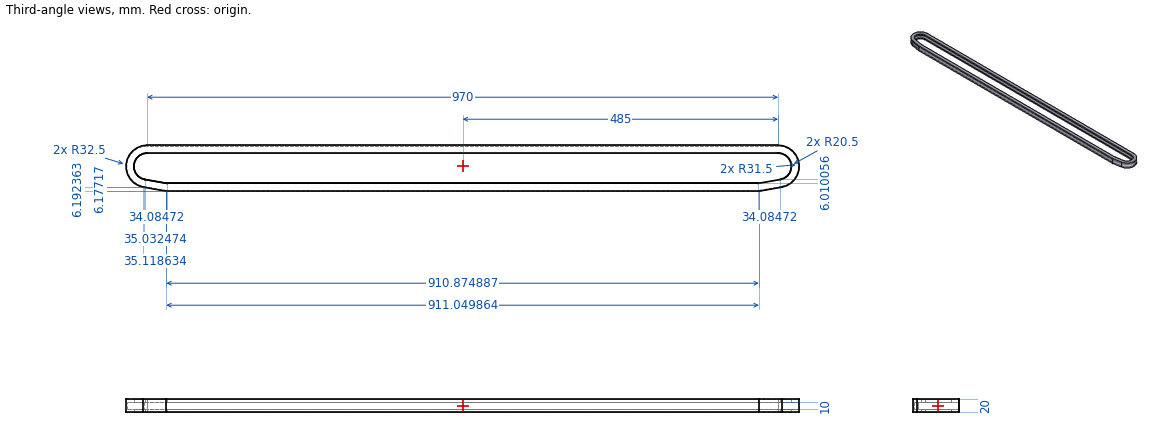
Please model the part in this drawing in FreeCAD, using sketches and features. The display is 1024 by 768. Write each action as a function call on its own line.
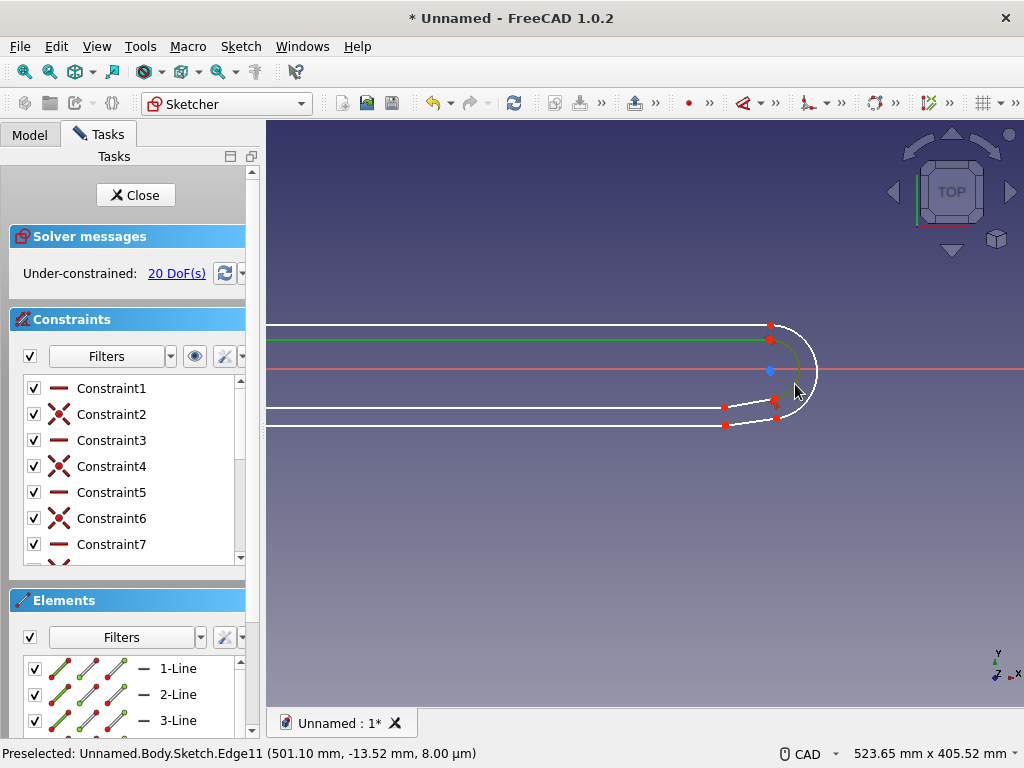
key(t)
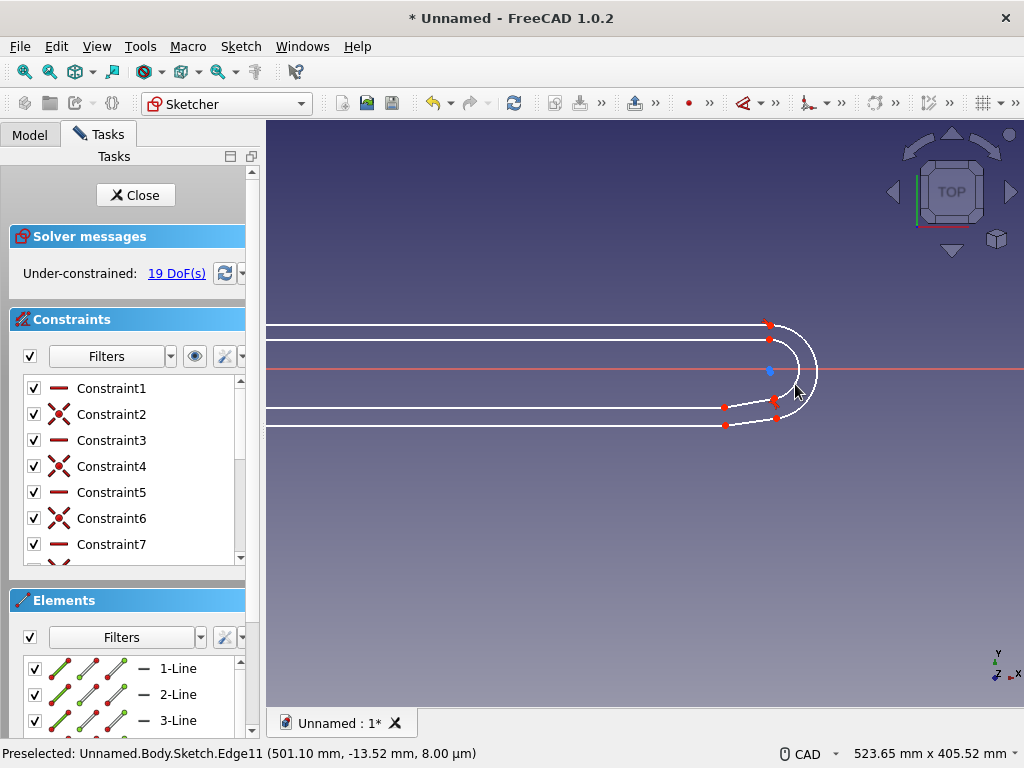
click(348, 340)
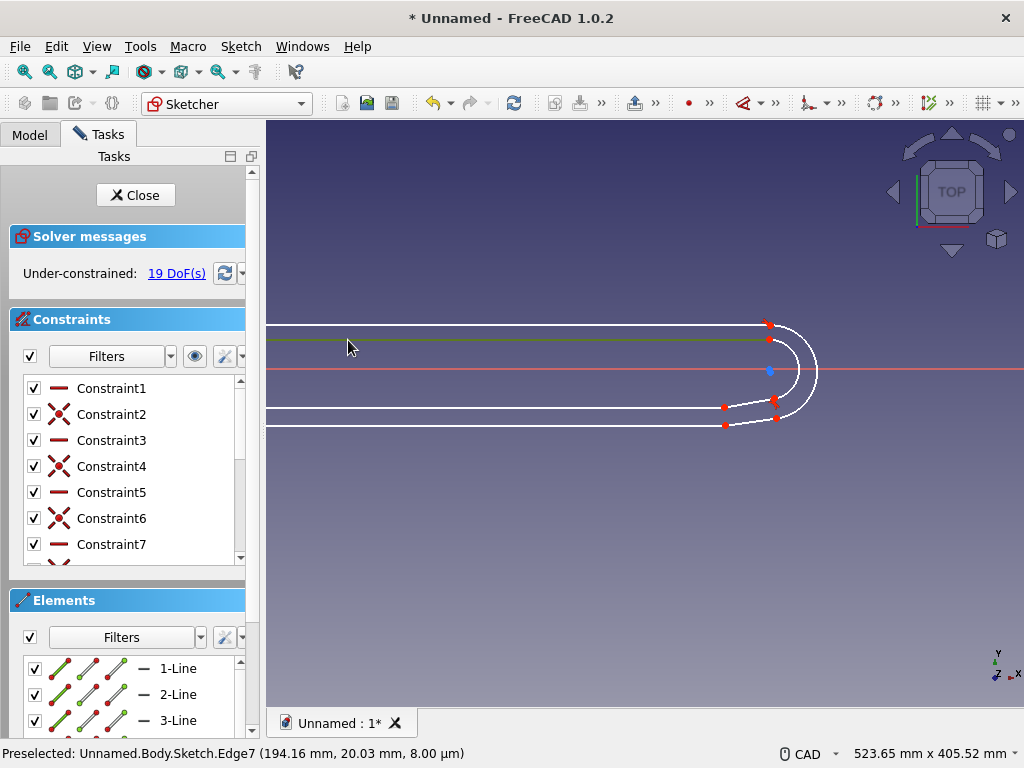
scroll(743, 427, down, 7)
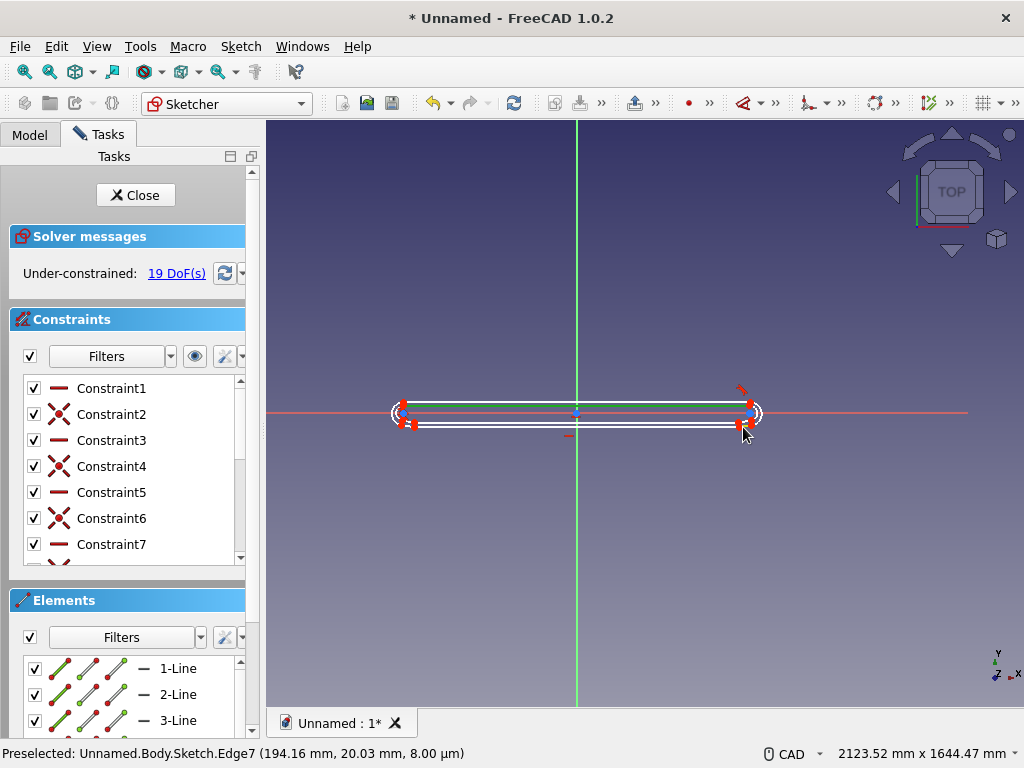
scroll(398, 409, up, 7)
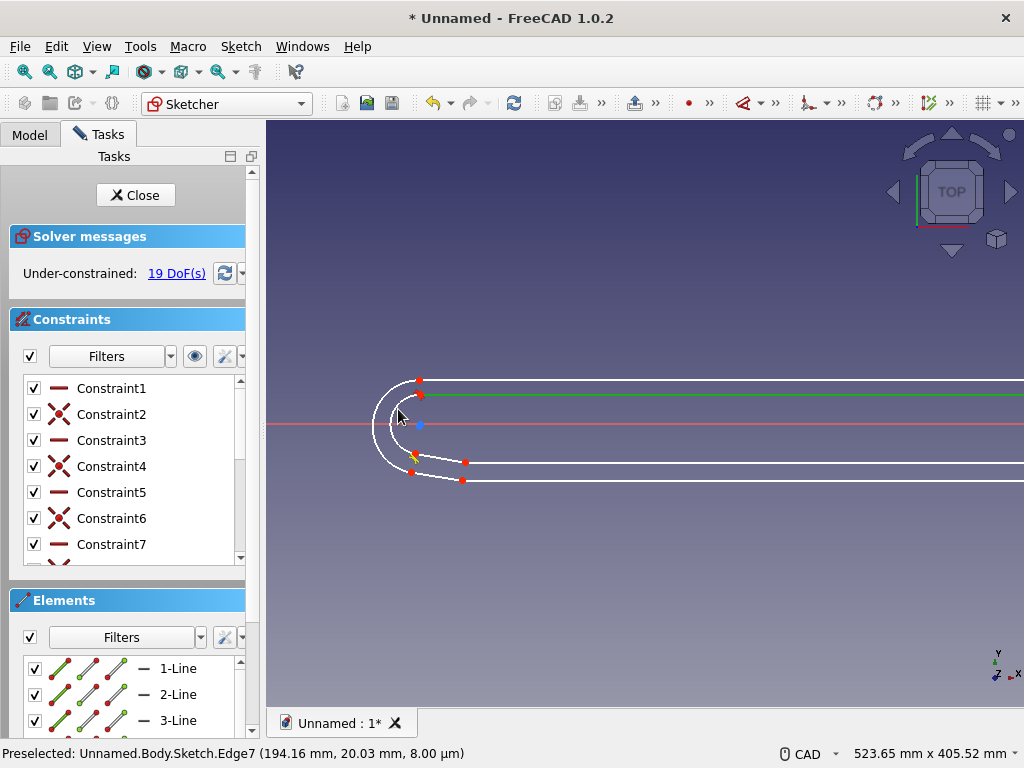
click(397, 406)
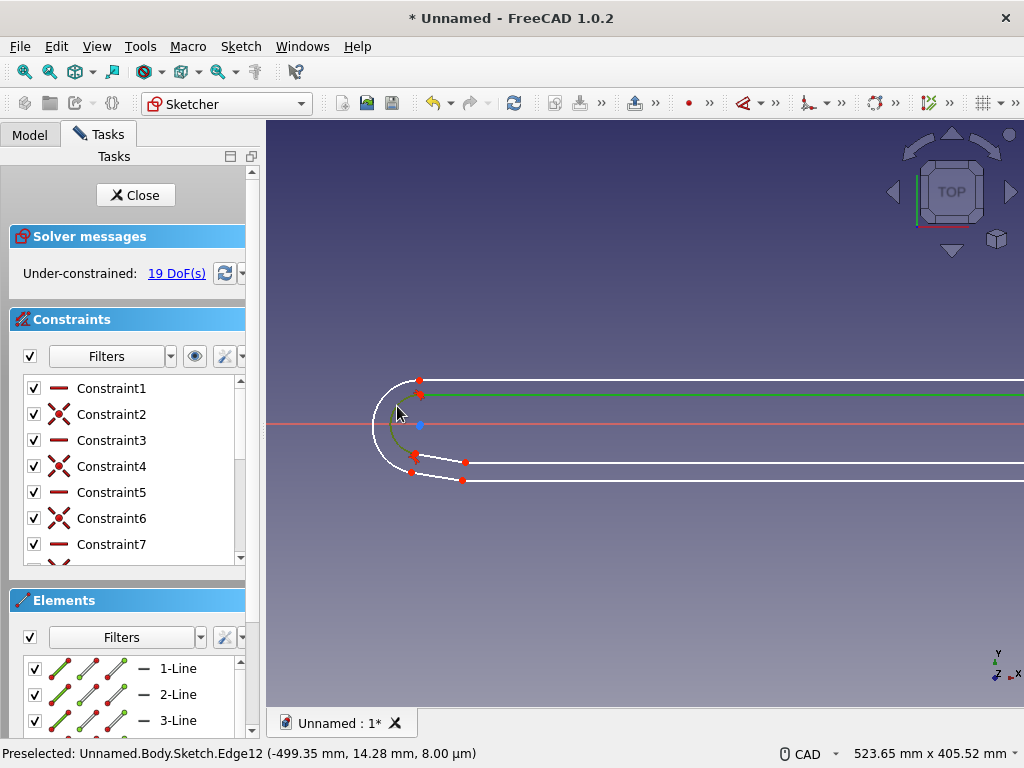
key(t)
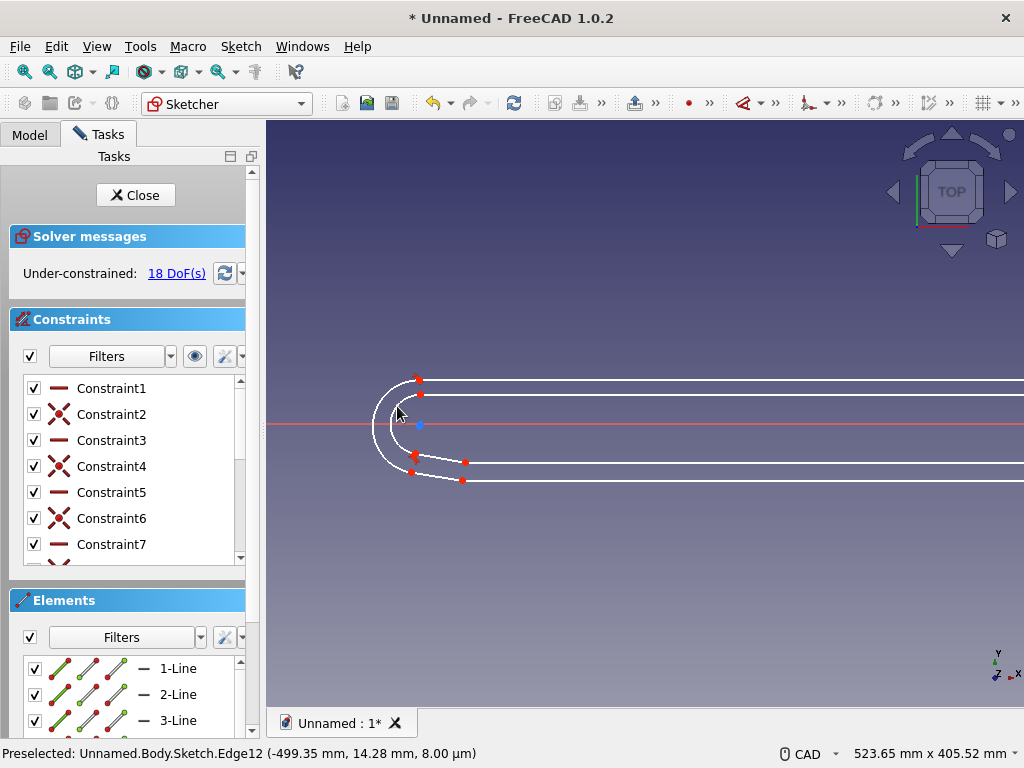
scroll(398, 409, down, 7)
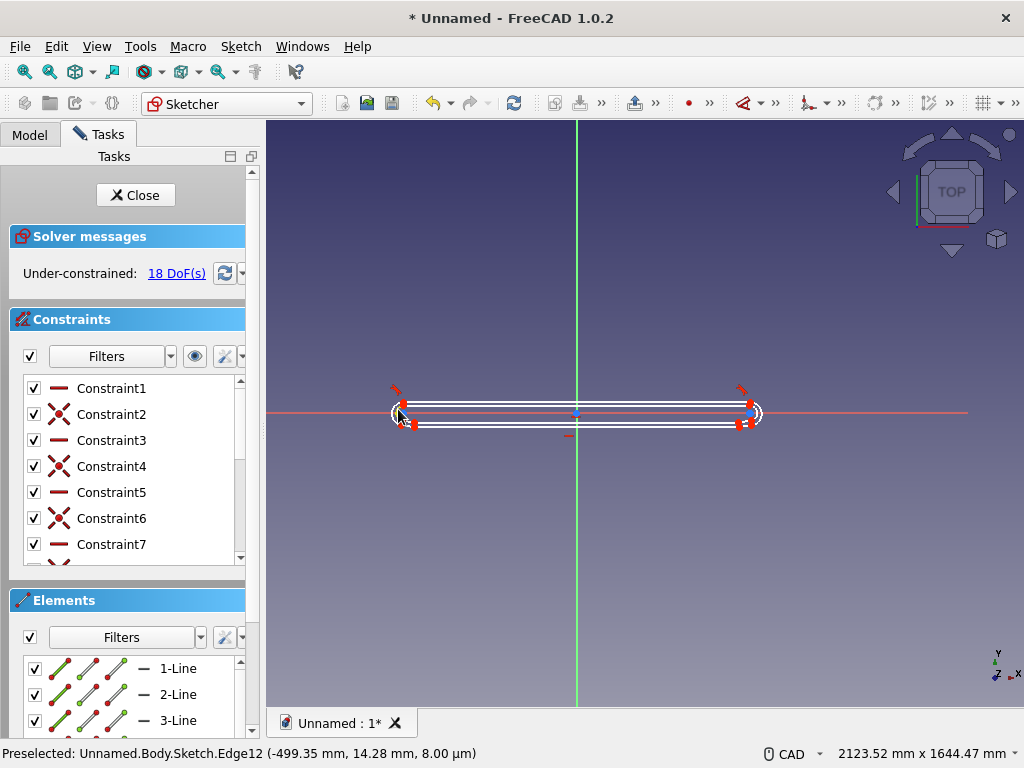
scroll(748, 421, up, 7)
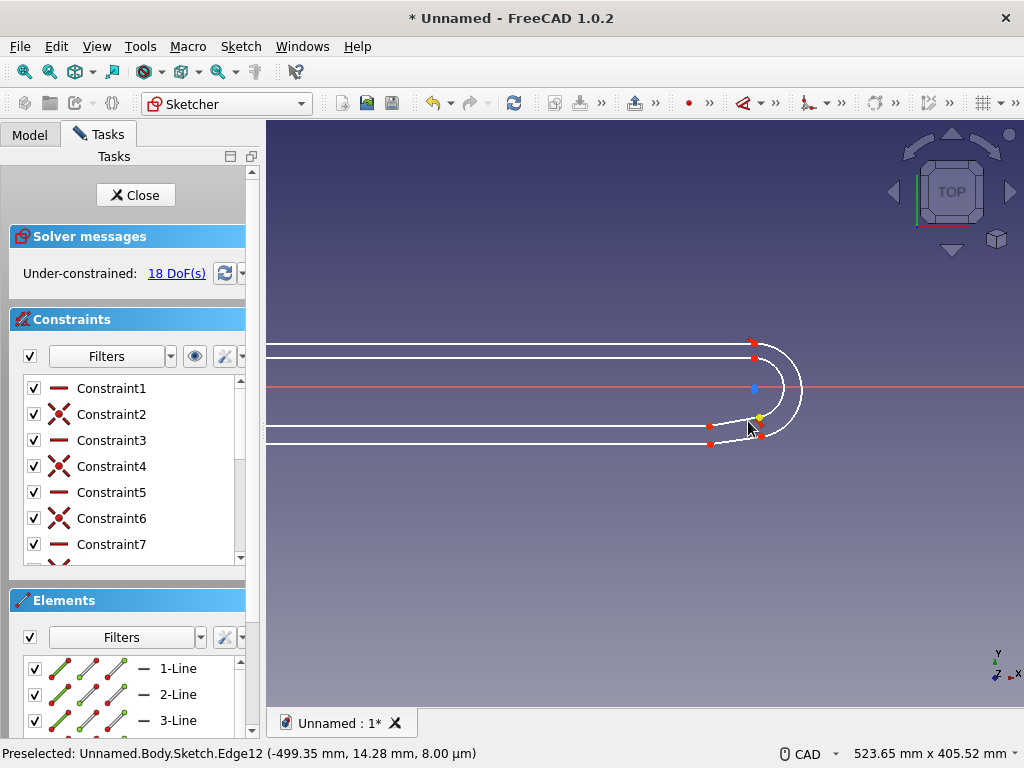
click(744, 420)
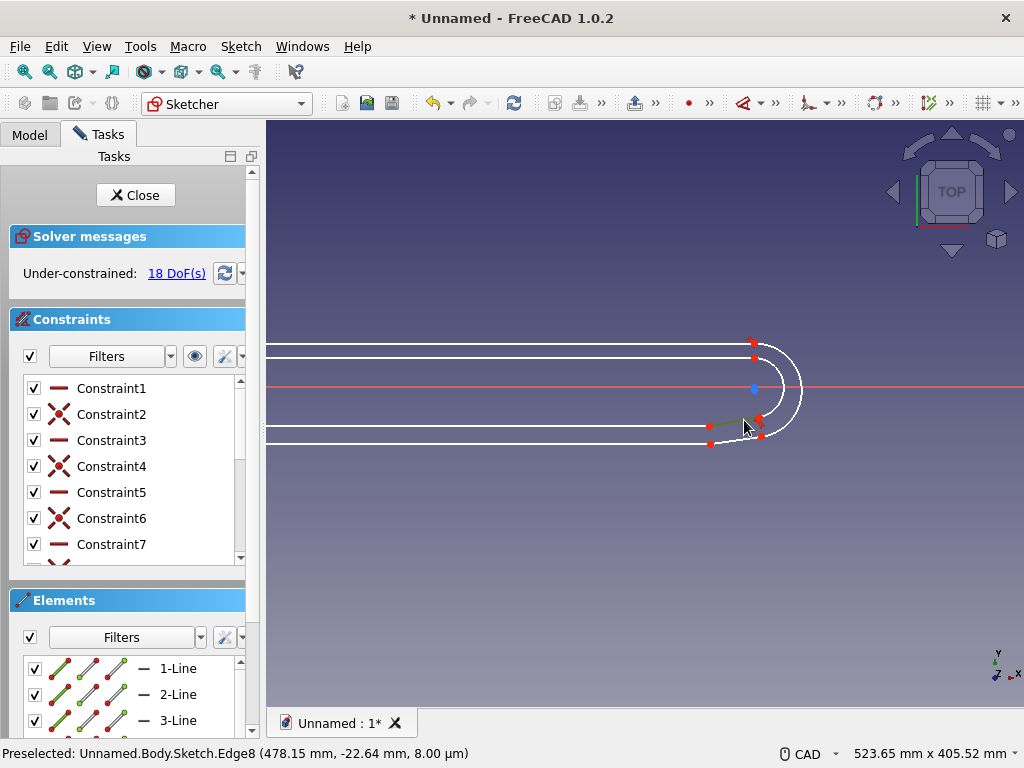
click(780, 402)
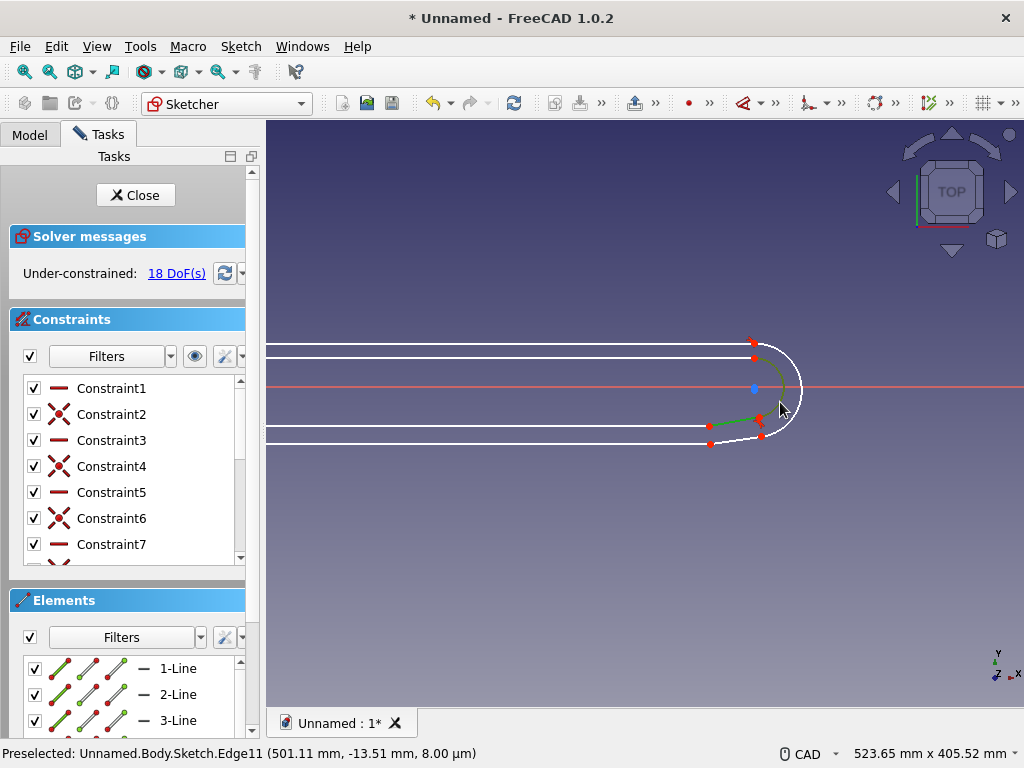
key(t)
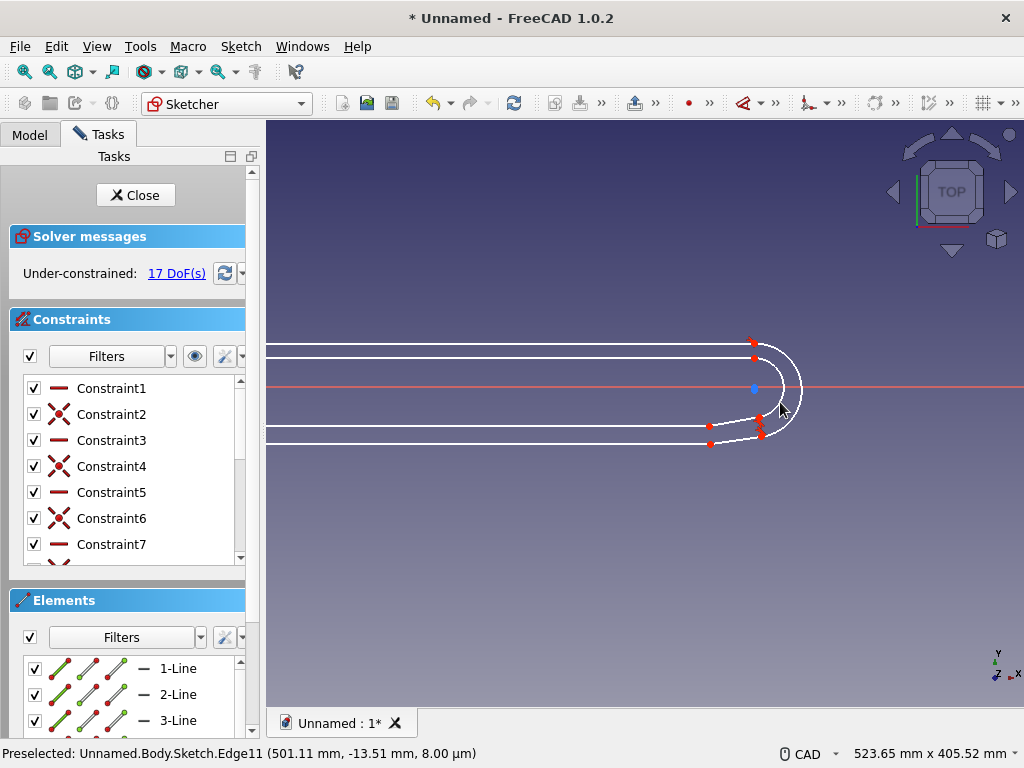
scroll(748, 421, down, 7)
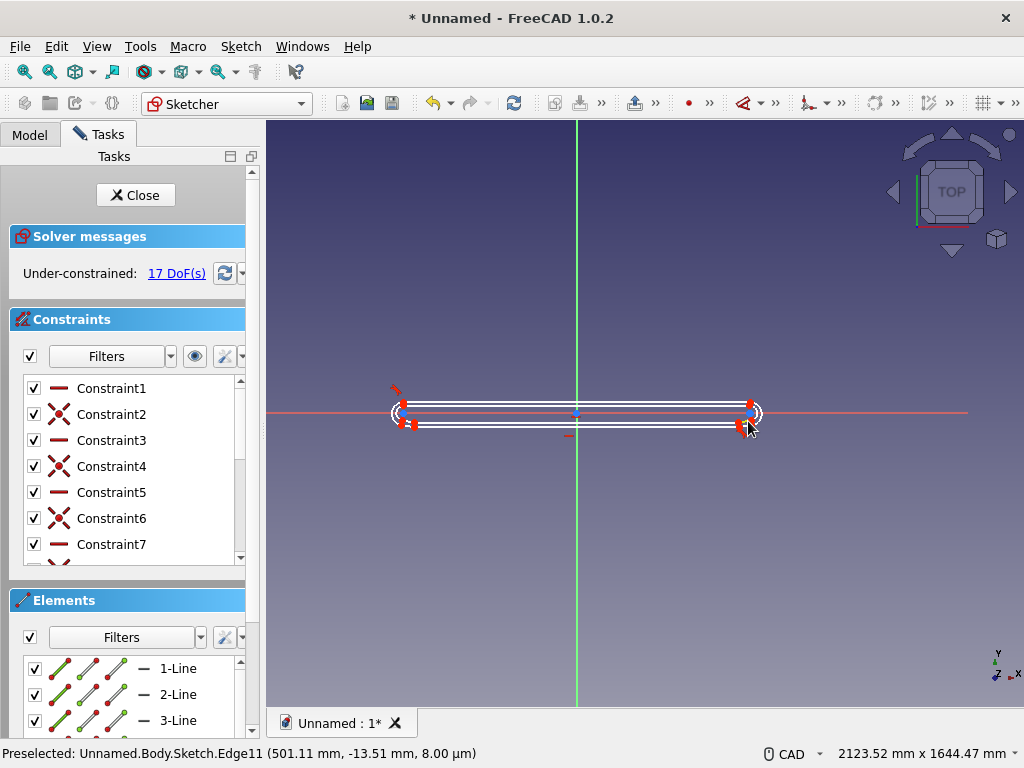
scroll(411, 422, up, 7)